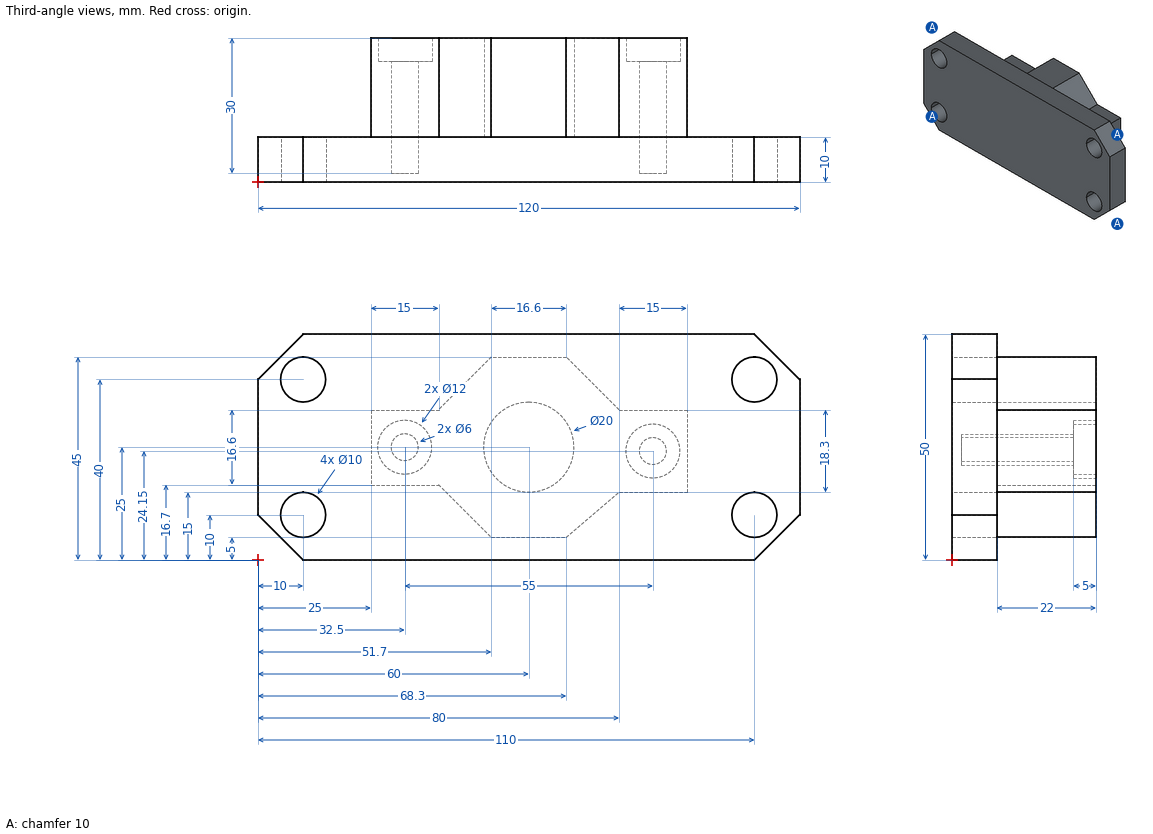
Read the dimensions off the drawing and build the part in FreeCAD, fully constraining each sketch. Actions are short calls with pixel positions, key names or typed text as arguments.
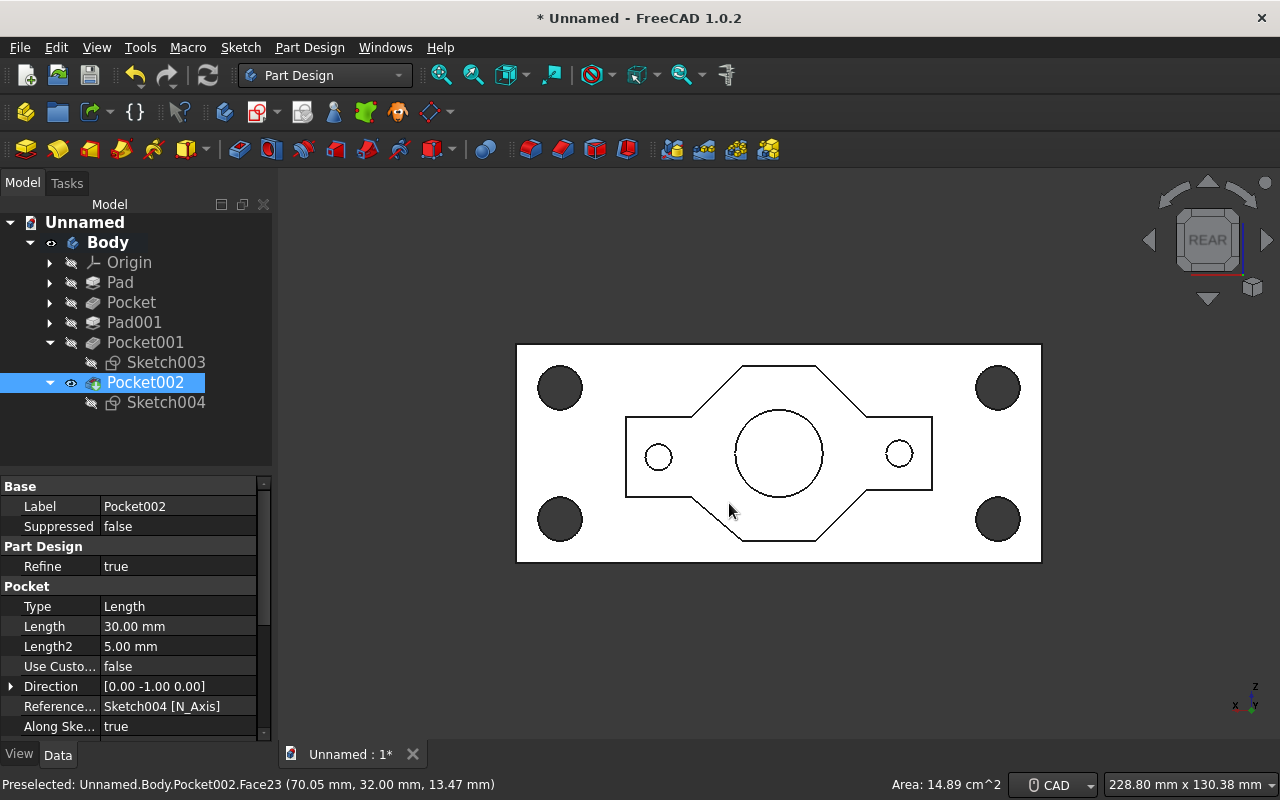
click(258, 112)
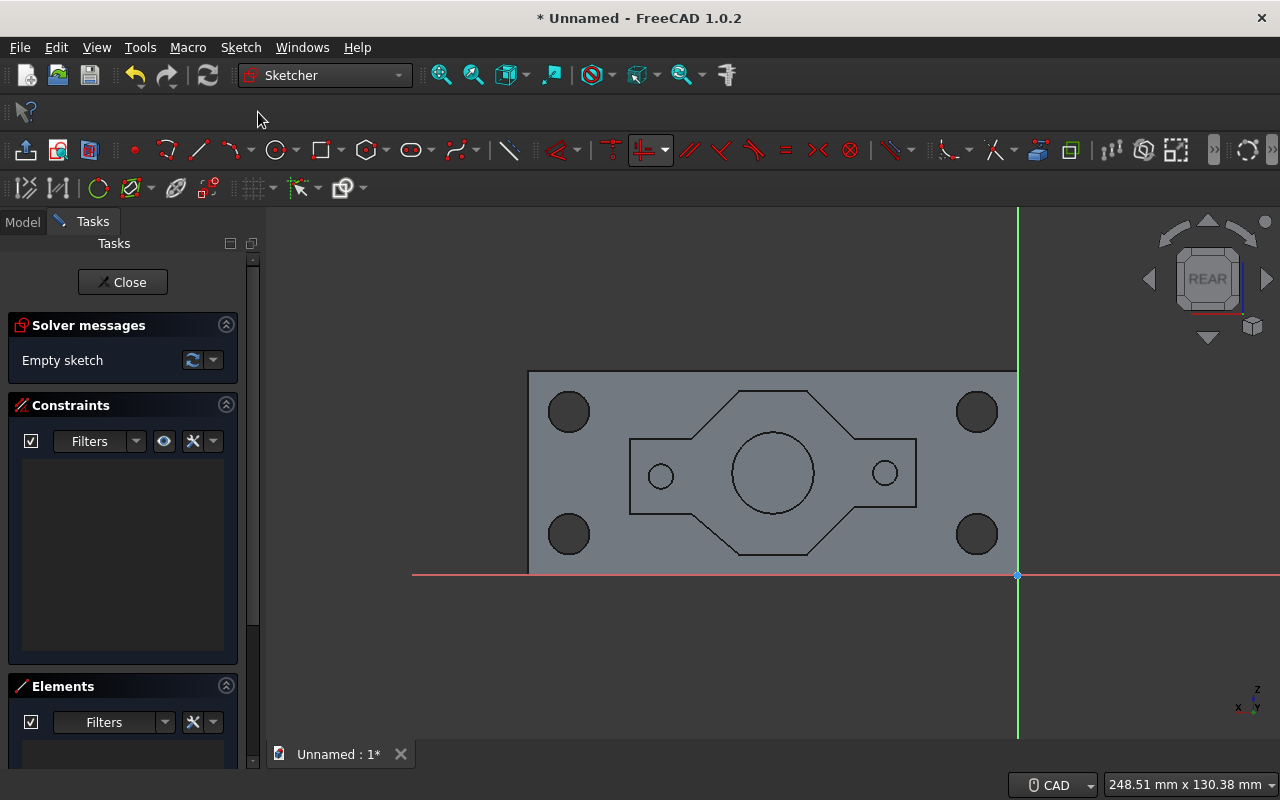
scroll(1076, 591, up, 2)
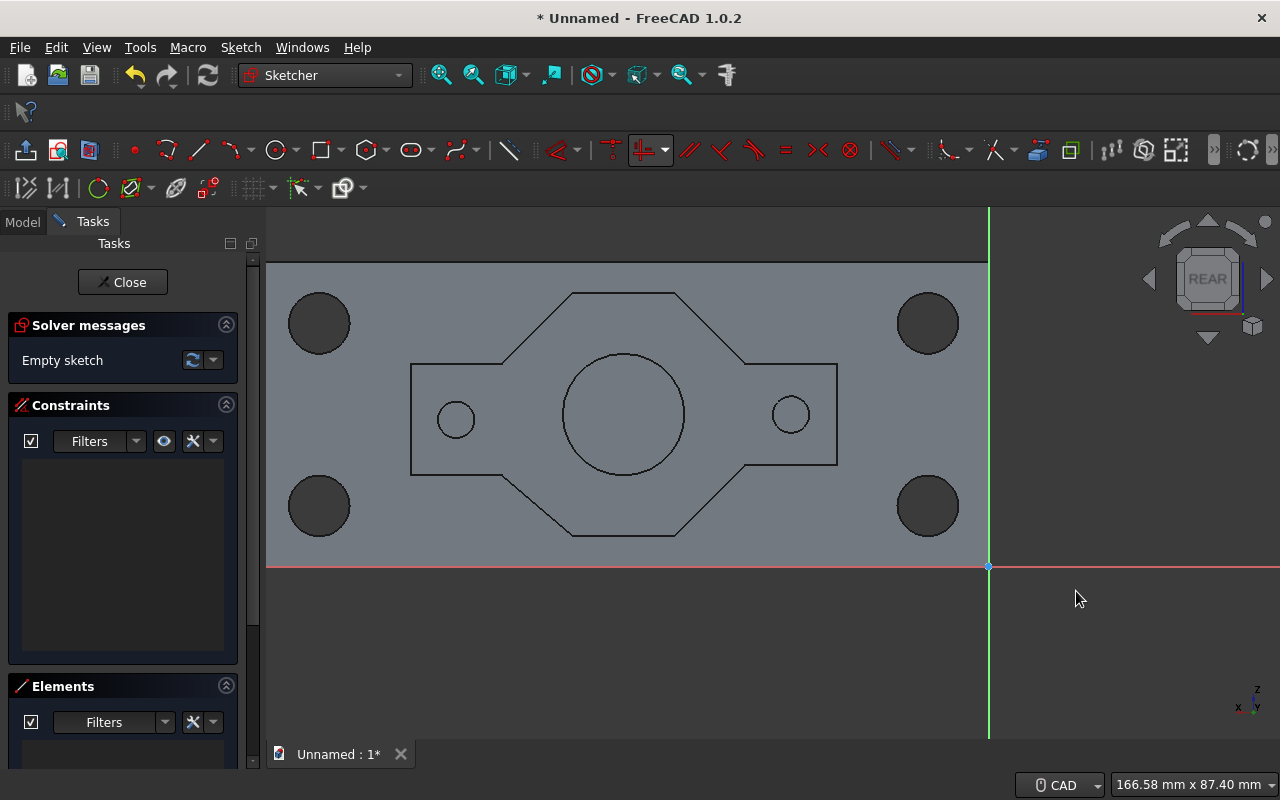
click(276, 150)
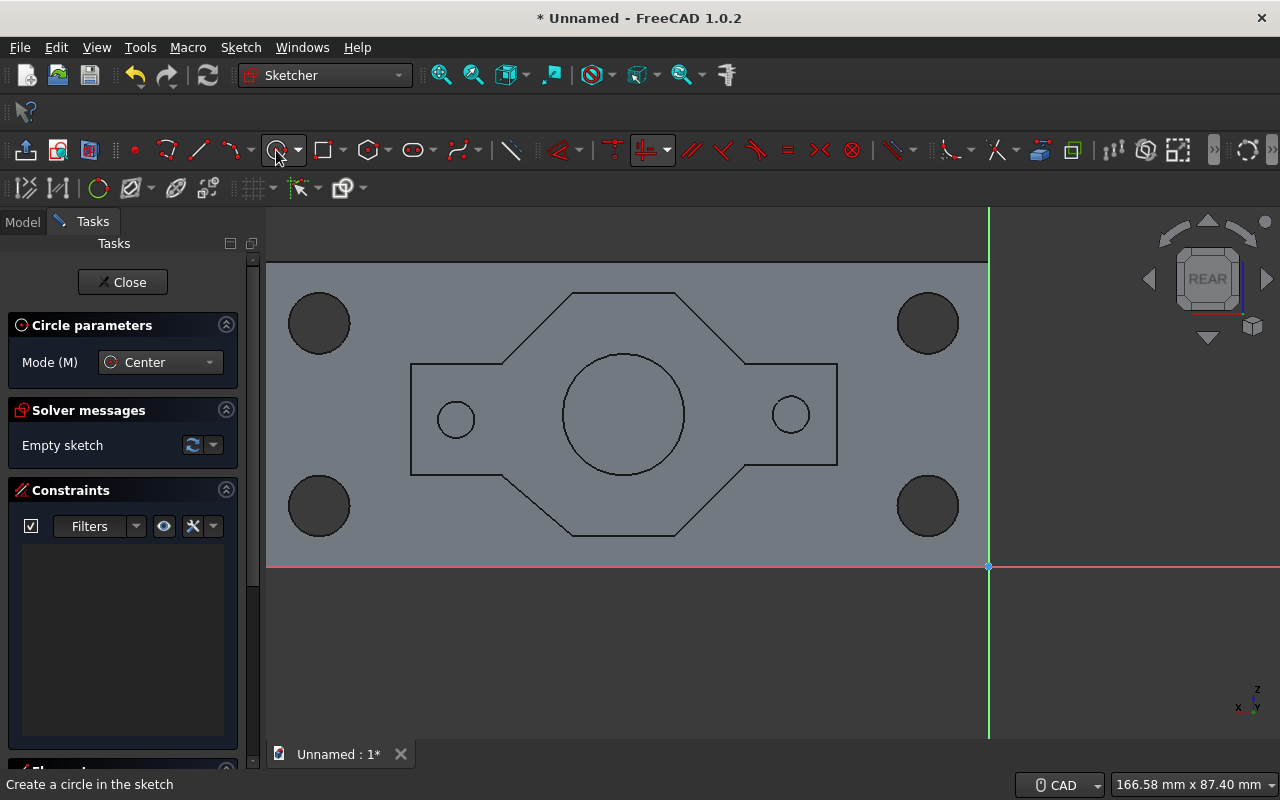
click(791, 415)
click(817, 389)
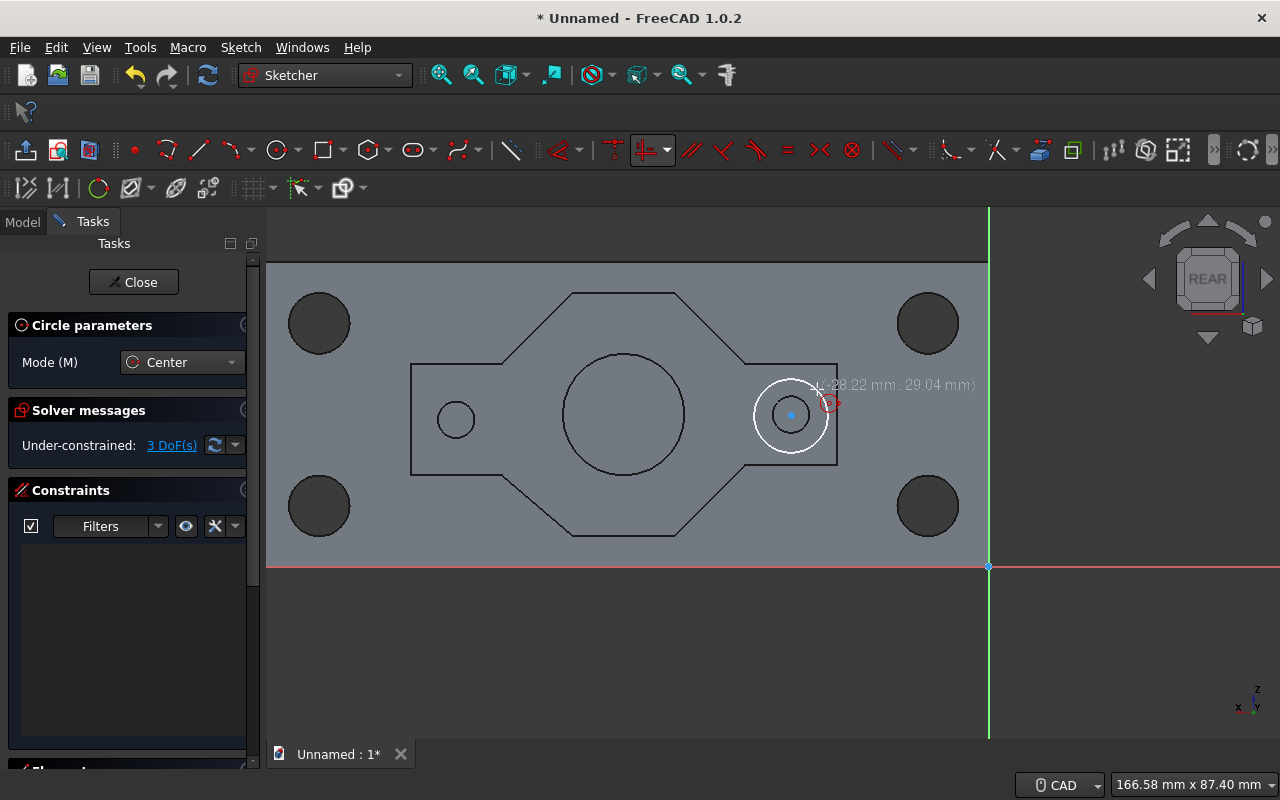
click(456, 420)
click(482, 394)
key(Escape)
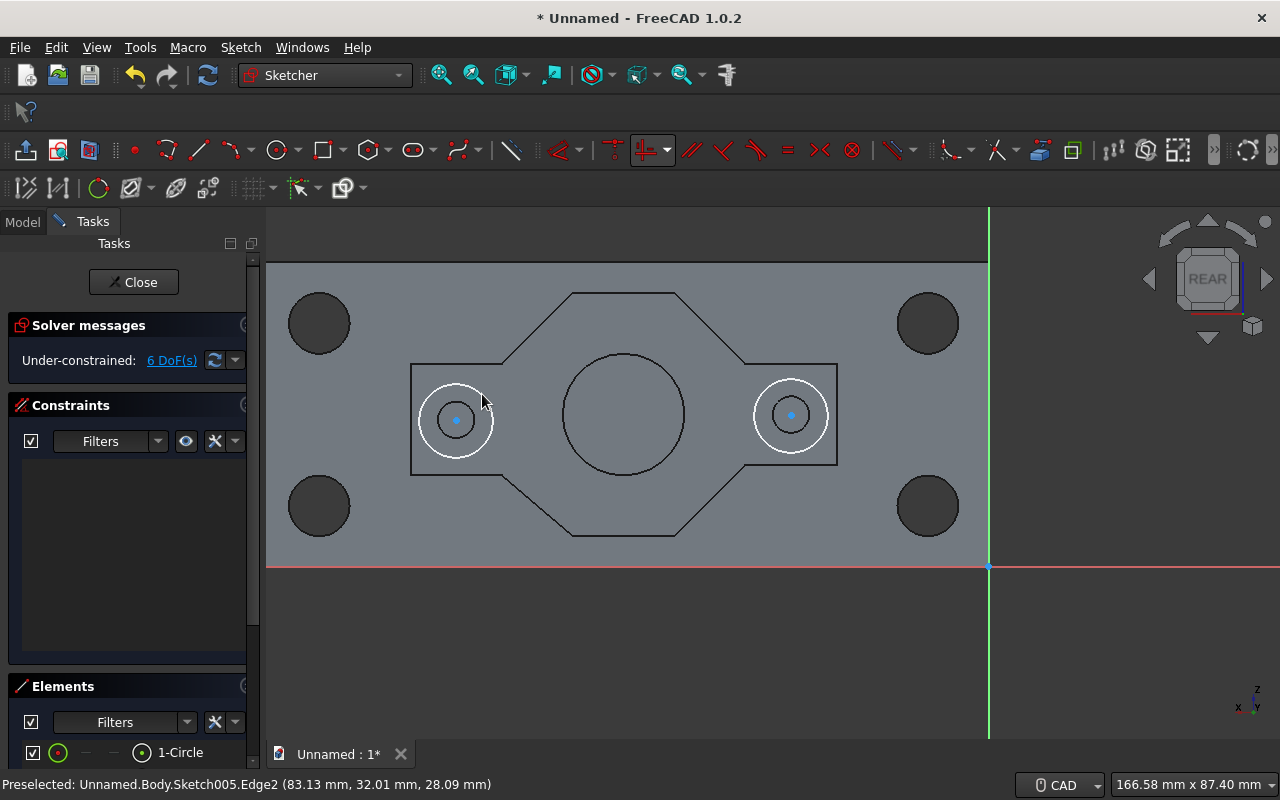
click(817, 390)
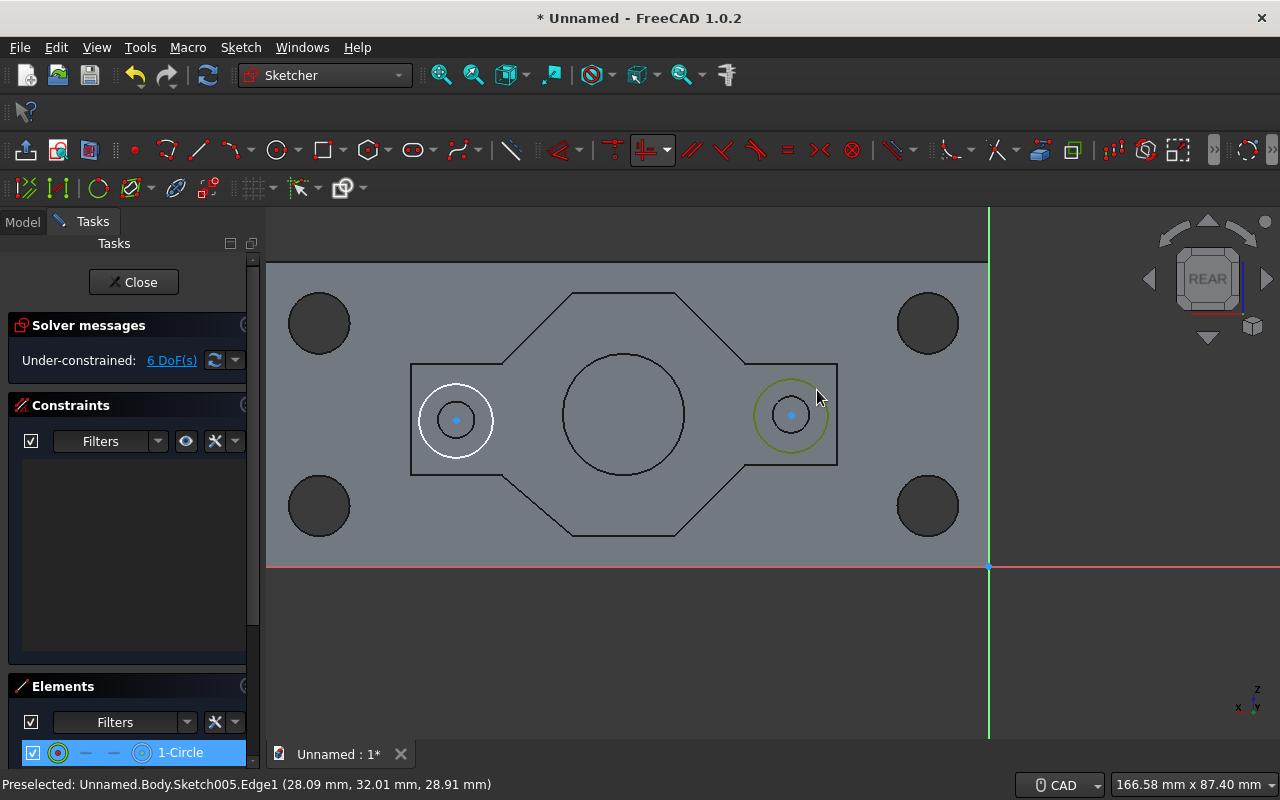
click(482, 395)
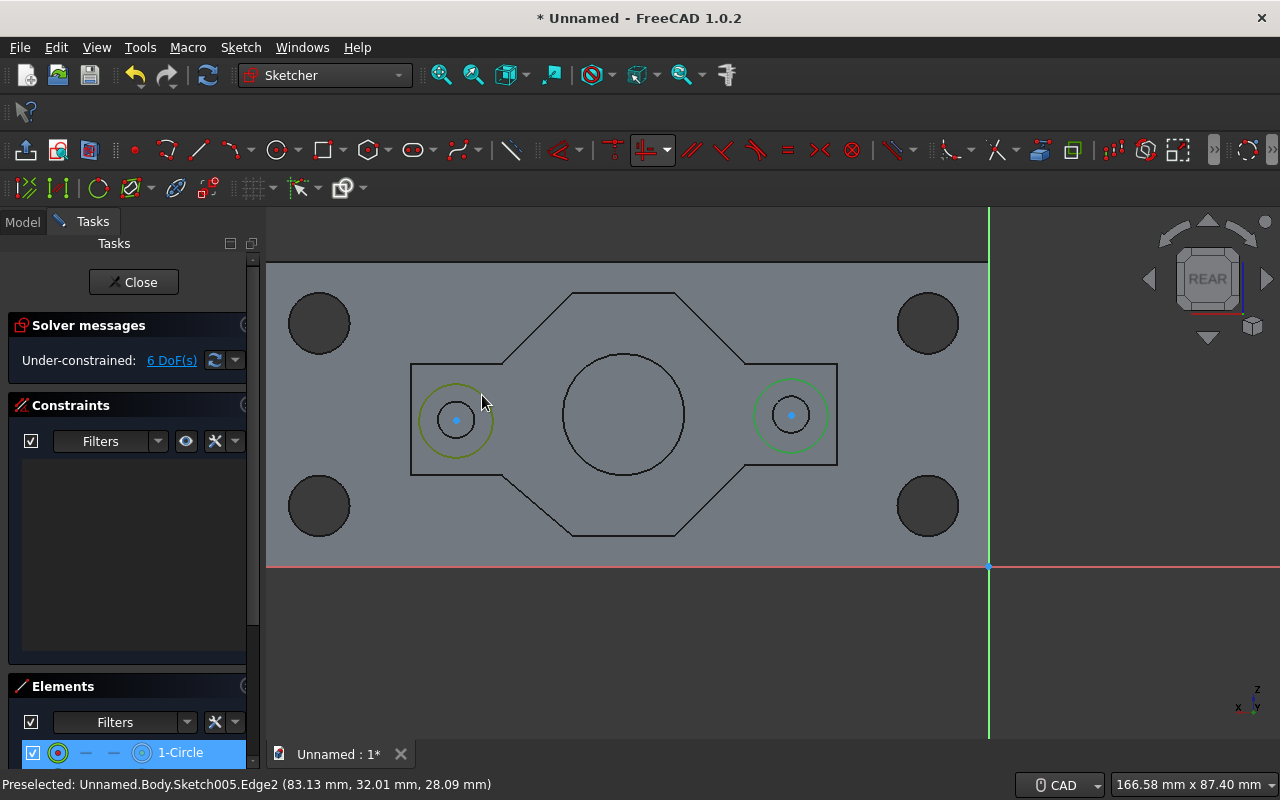
click(788, 150)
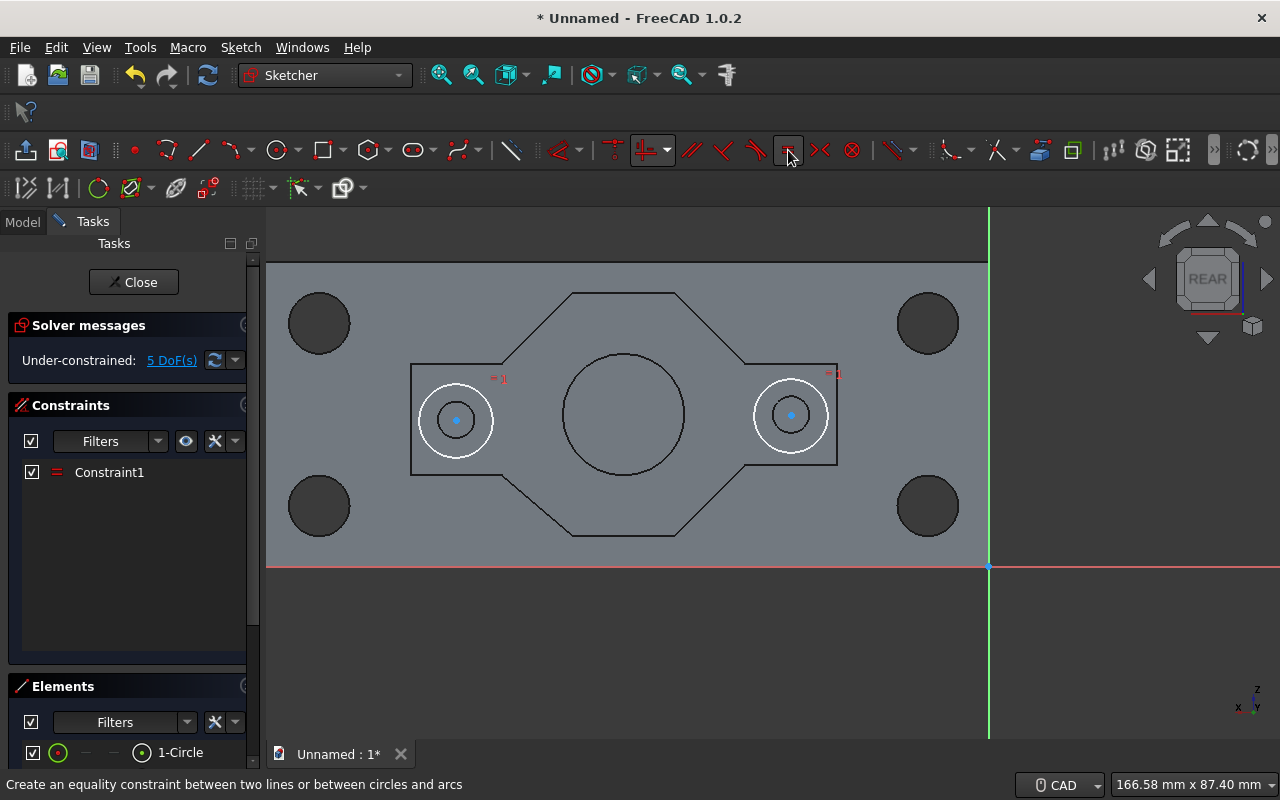
click(558, 150)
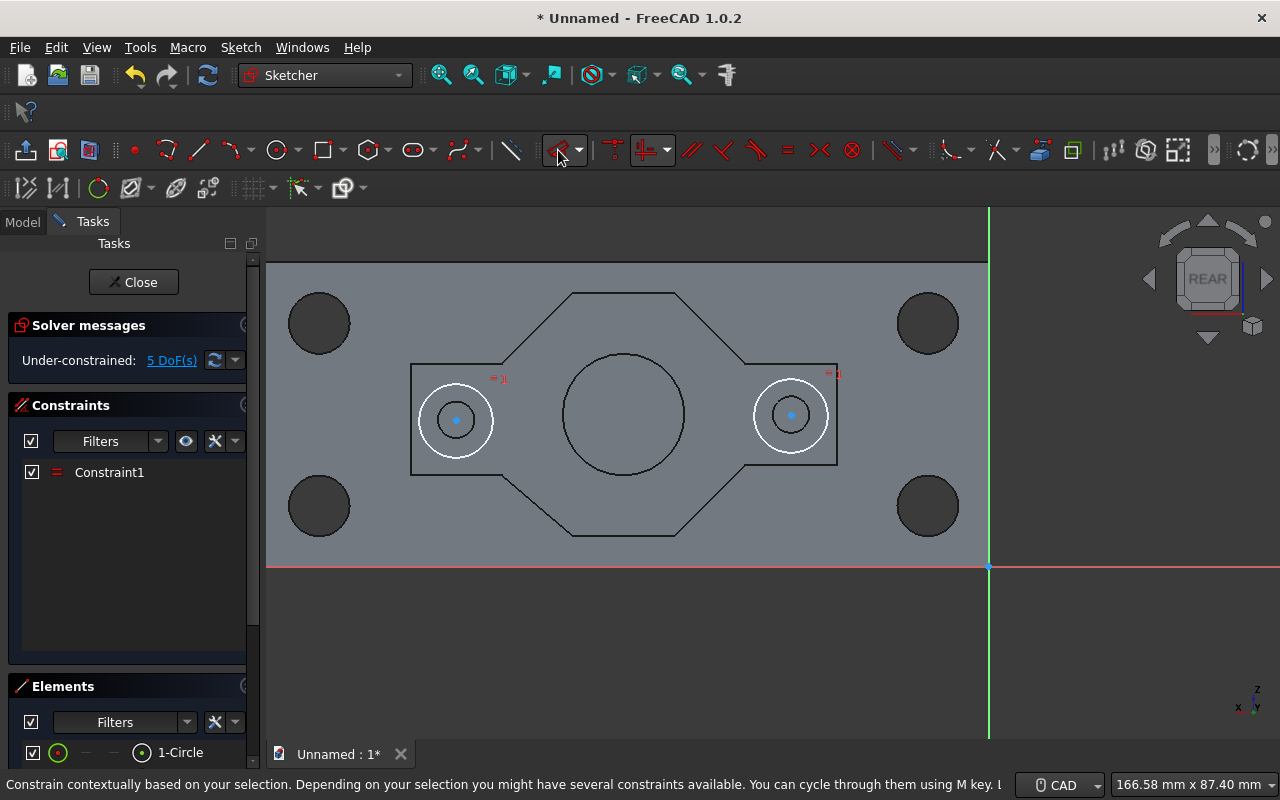
click(817, 390)
click(840, 367)